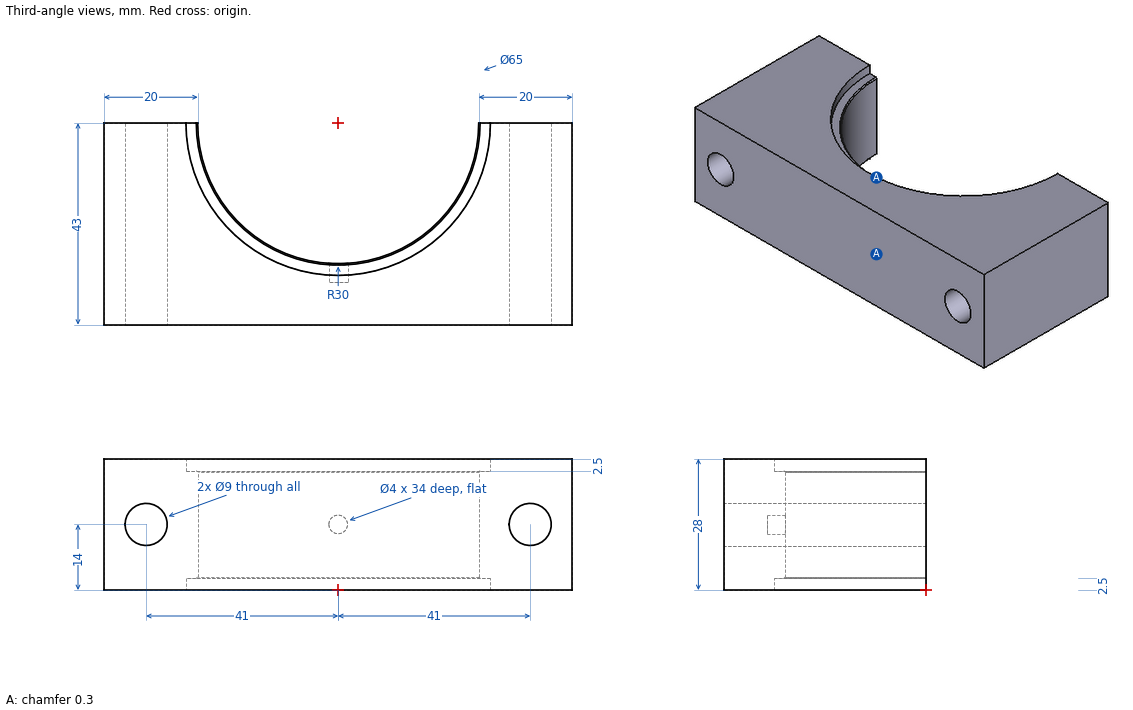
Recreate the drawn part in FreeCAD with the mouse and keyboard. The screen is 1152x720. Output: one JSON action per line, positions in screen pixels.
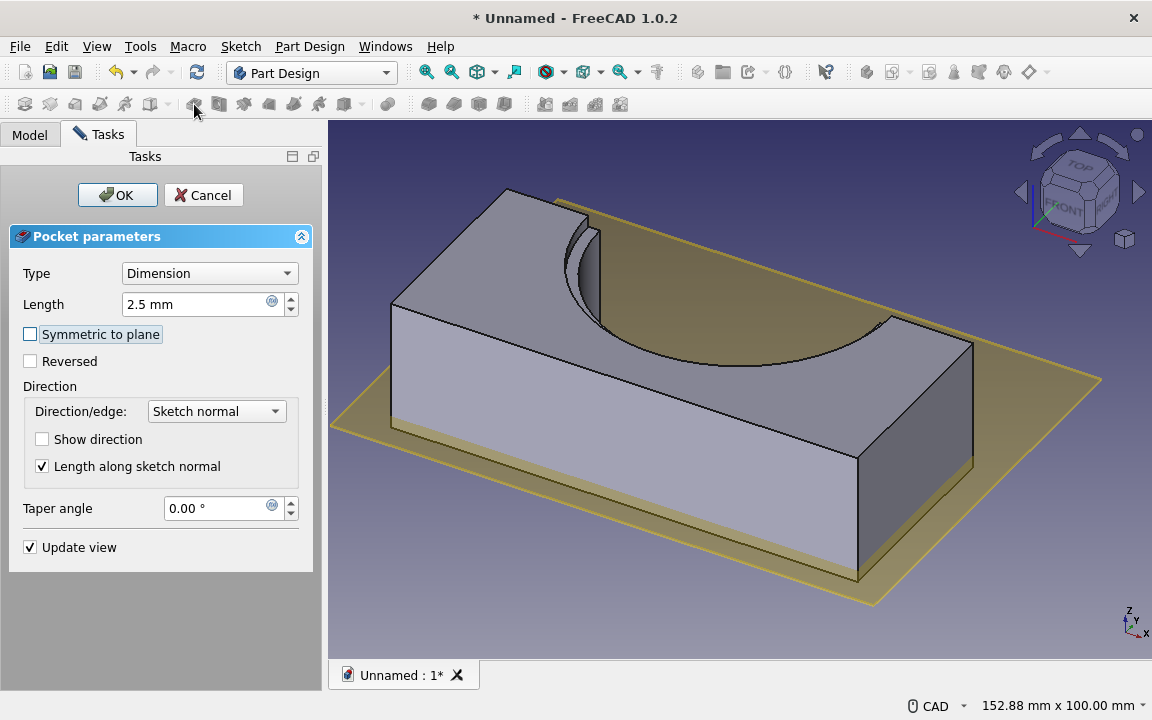
{"action": "left_click", "coordinate": [118, 195]}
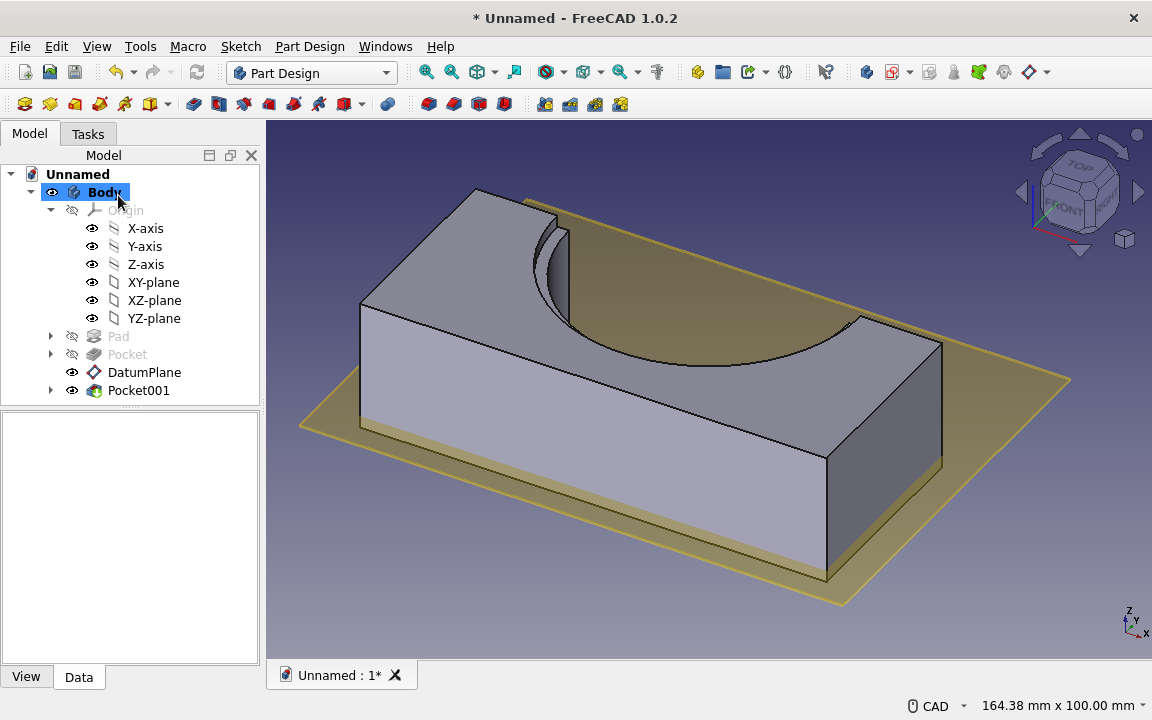
{"action": "left_click", "coordinate": [117, 372]}
{"action": "key", "text": "space"}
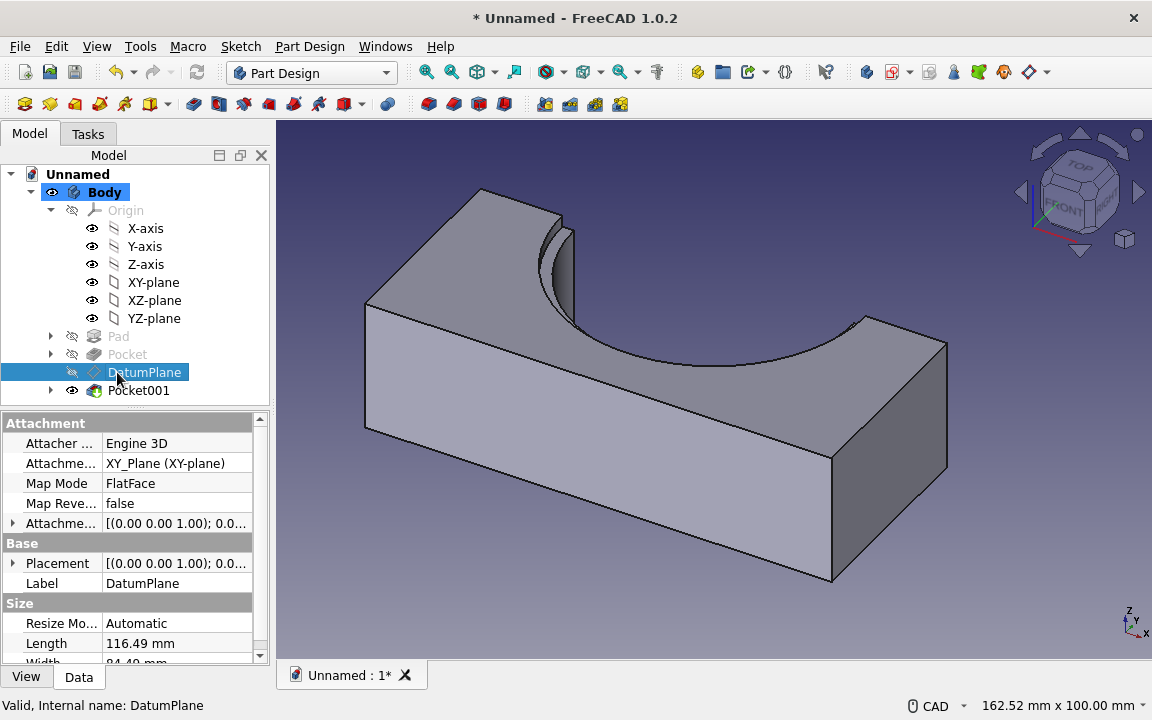
{"action": "left_click", "coordinate": [554, 262]}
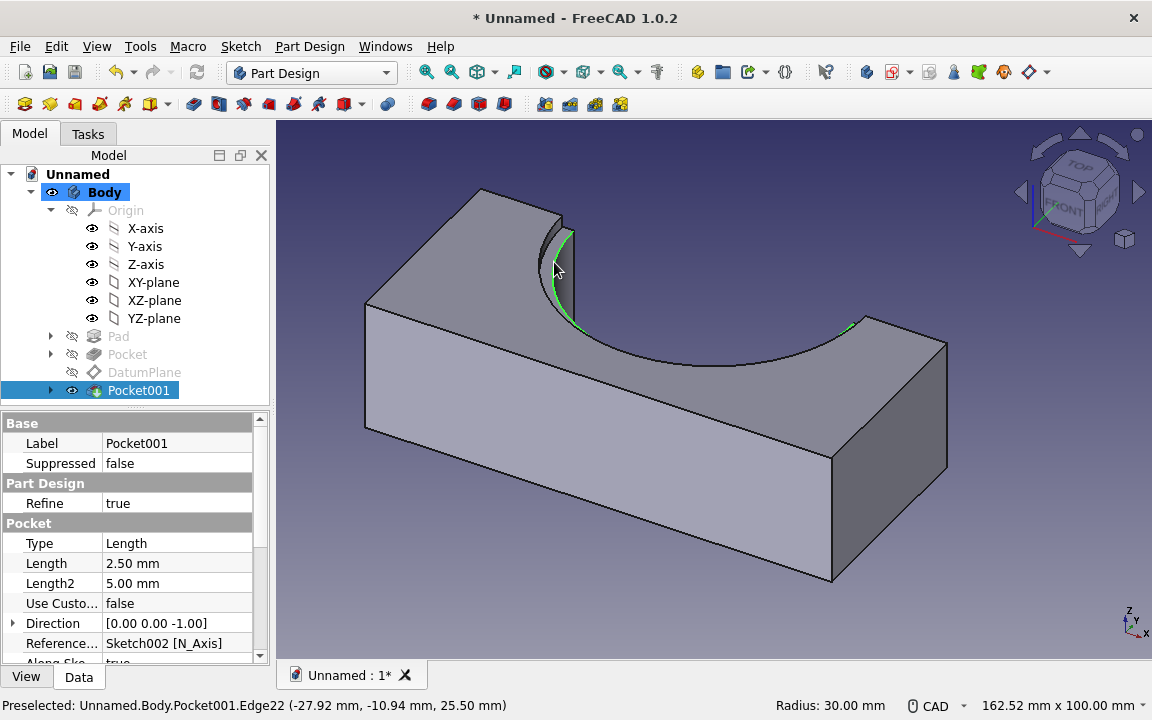
{"action": "key", "text": "0"}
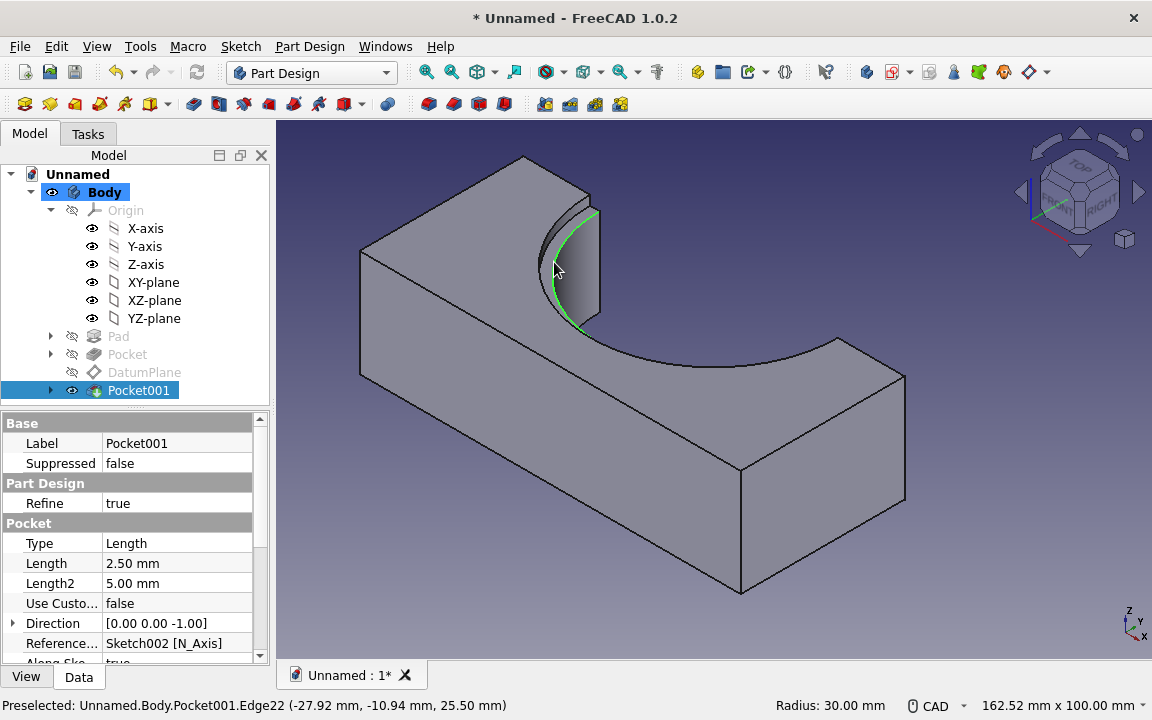
{"action": "key", "text": "2"}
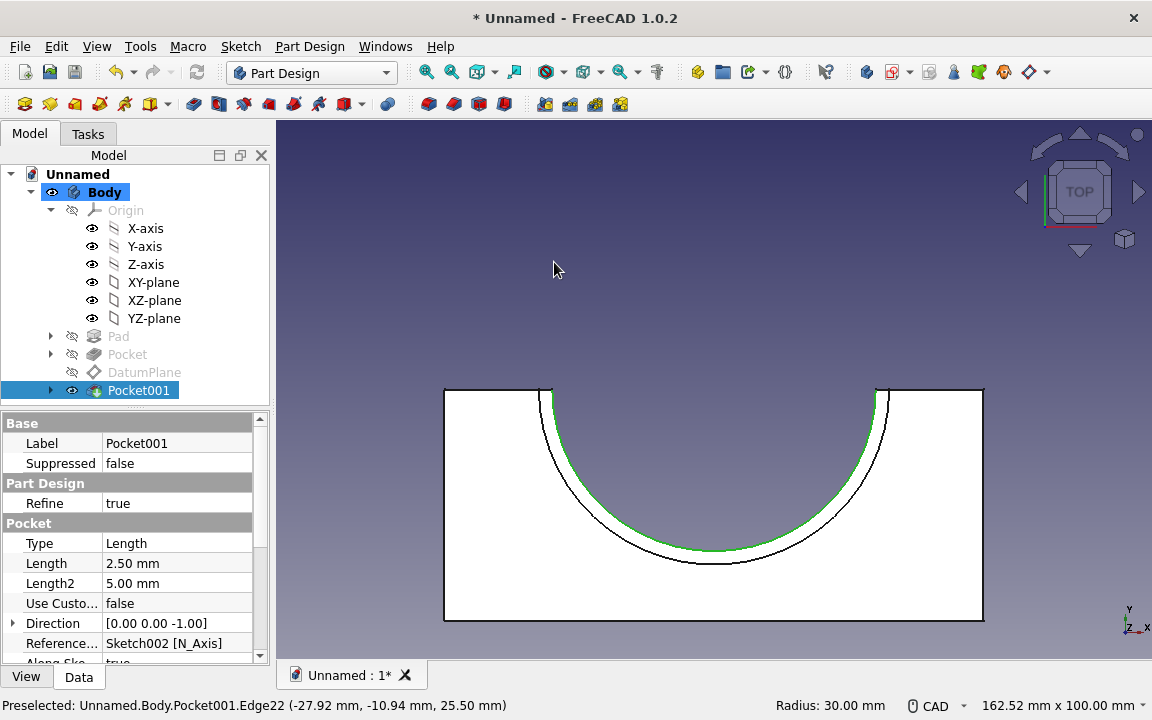
{"action": "key", "text": "1"}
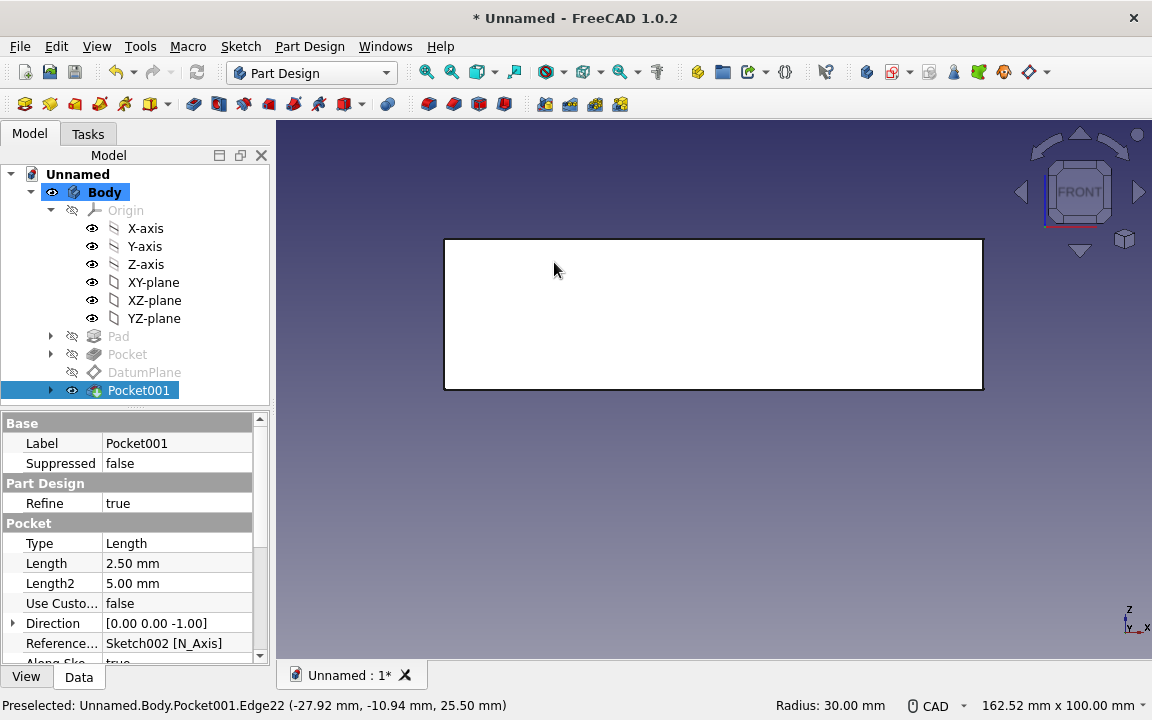
{"action": "key", "text": "3"}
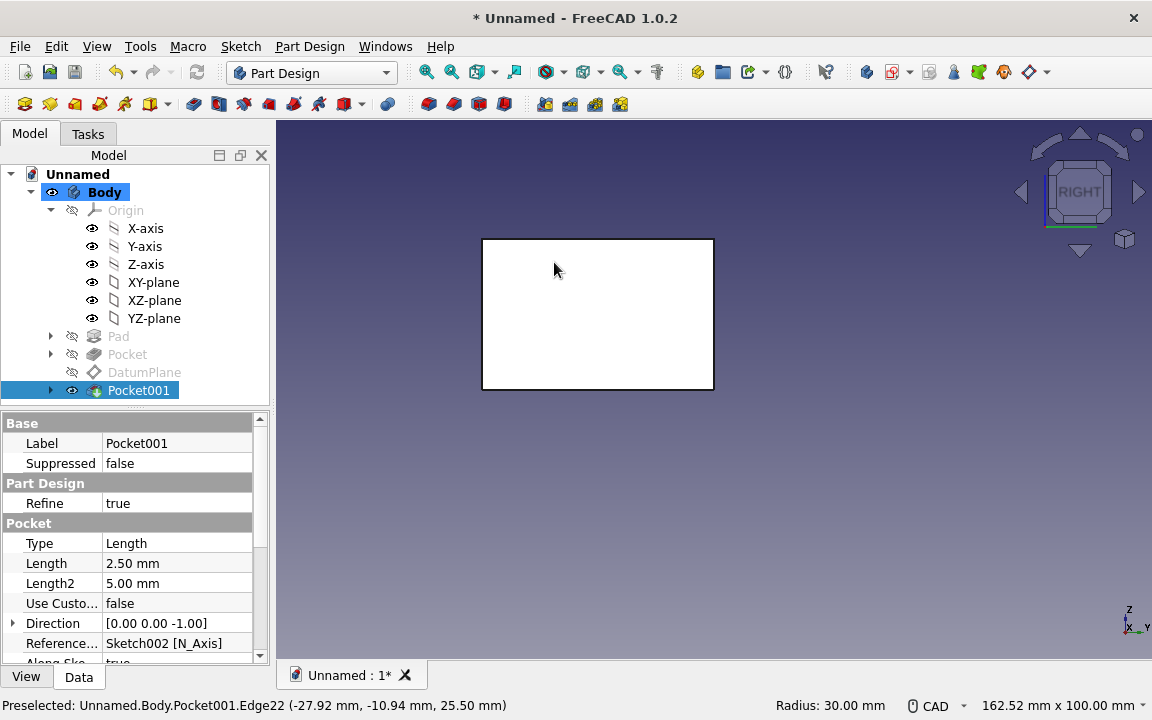
{"action": "left_click", "coordinate": [427, 72]}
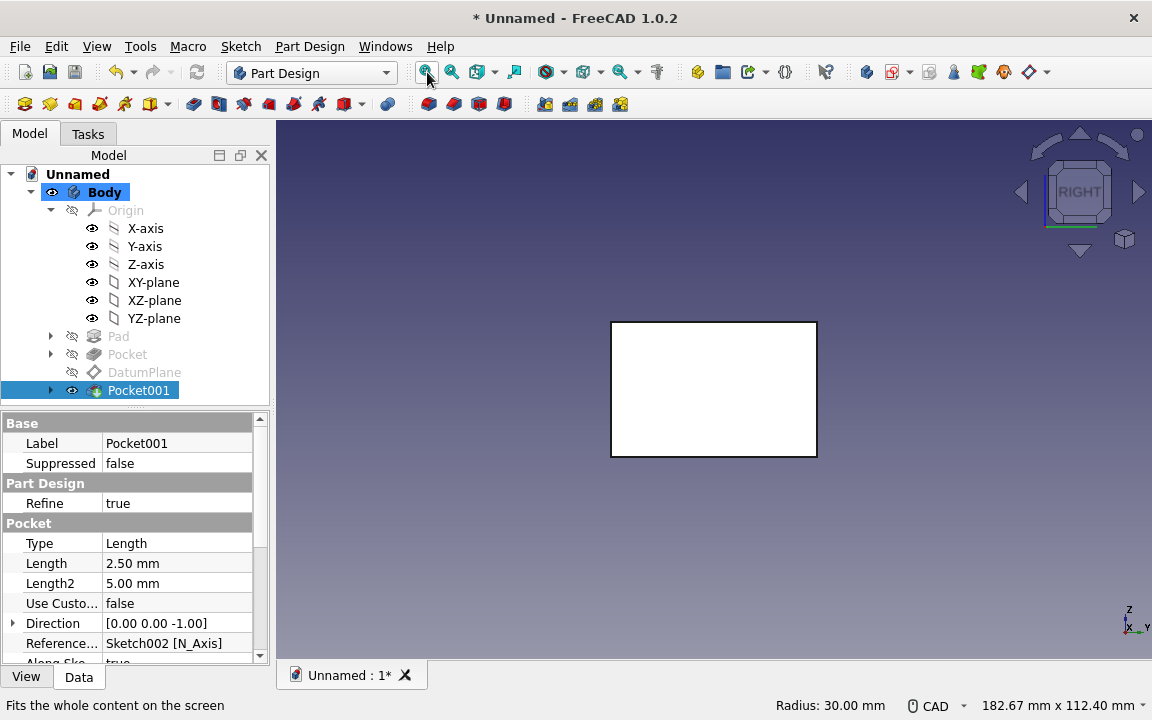
{"action": "key", "text": "5"}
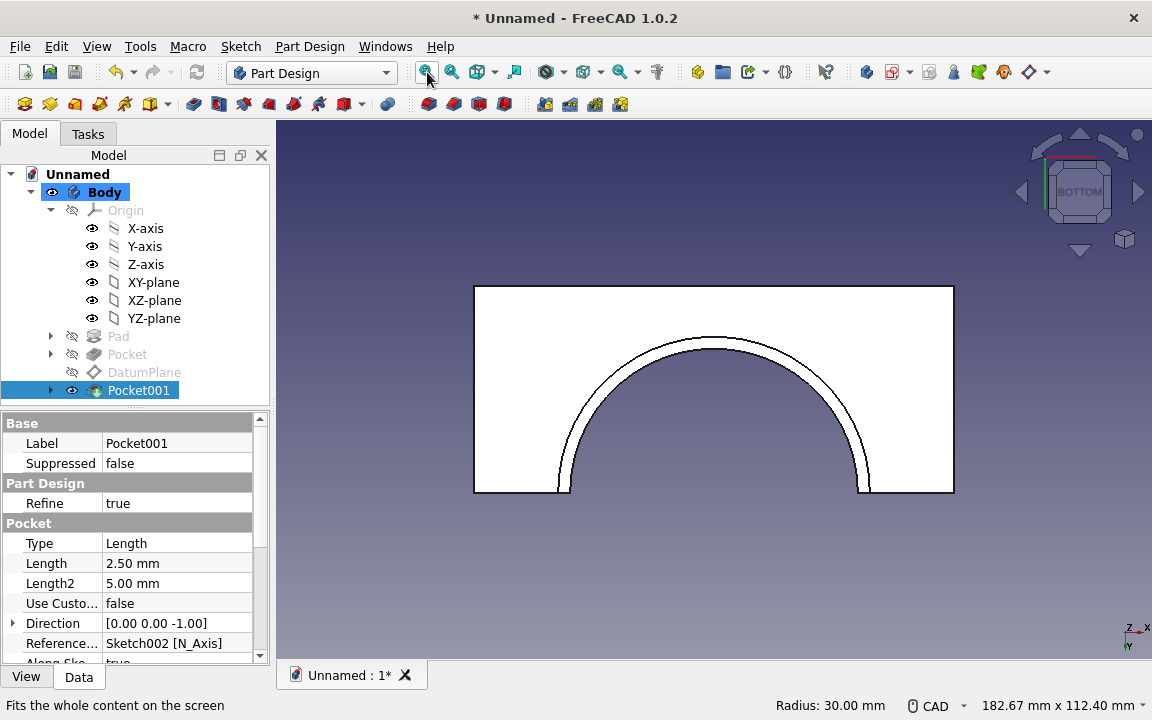
{"action": "left_click", "coordinate": [714, 348], "text": "ctrl"}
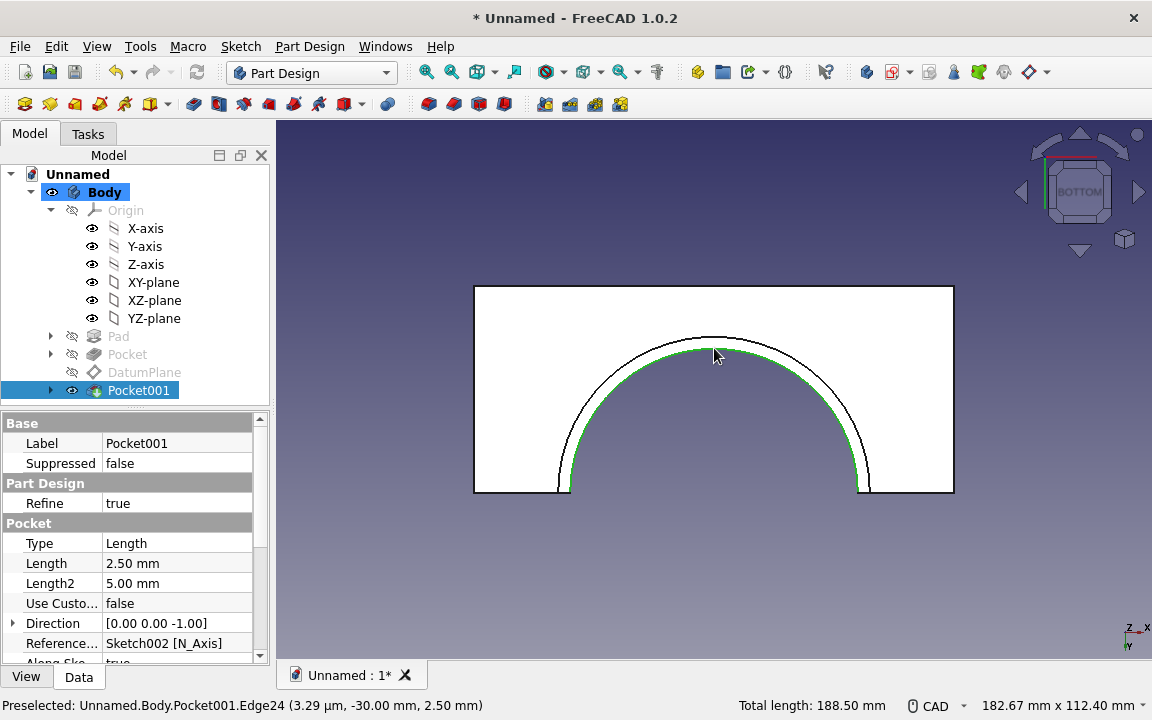
{"action": "left_click", "coordinate": [454, 104]}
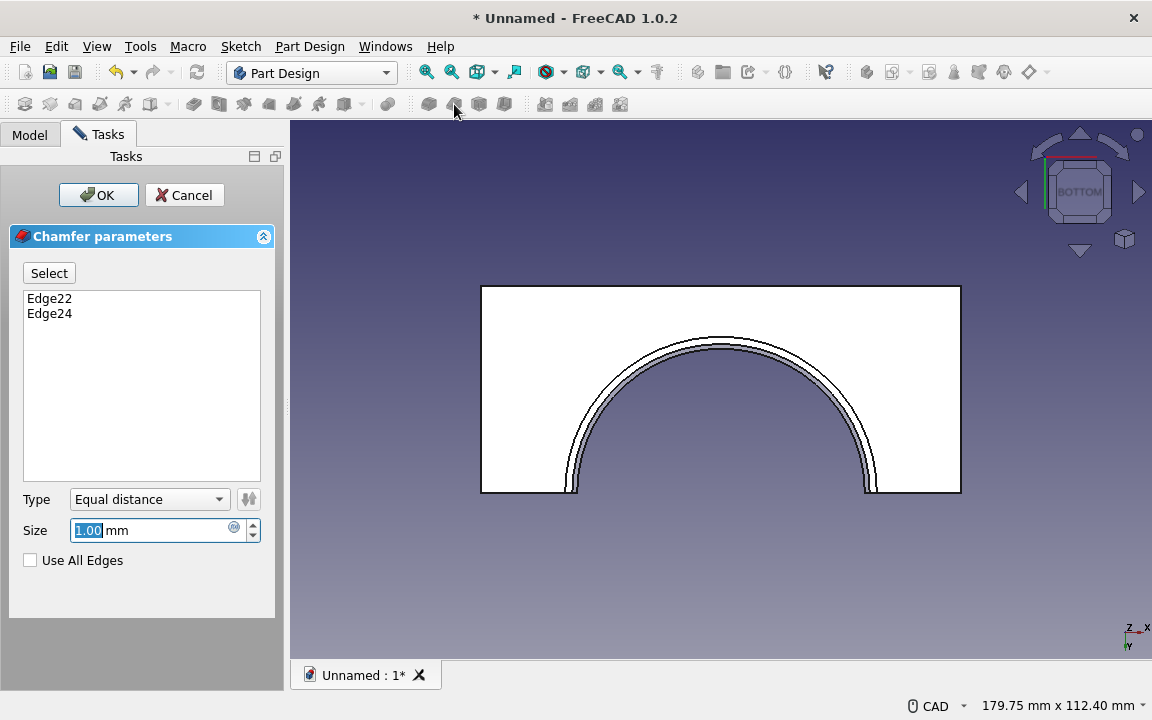
{"action": "type", "text": "0.3"}
{"action": "key", "text": "Tab"}